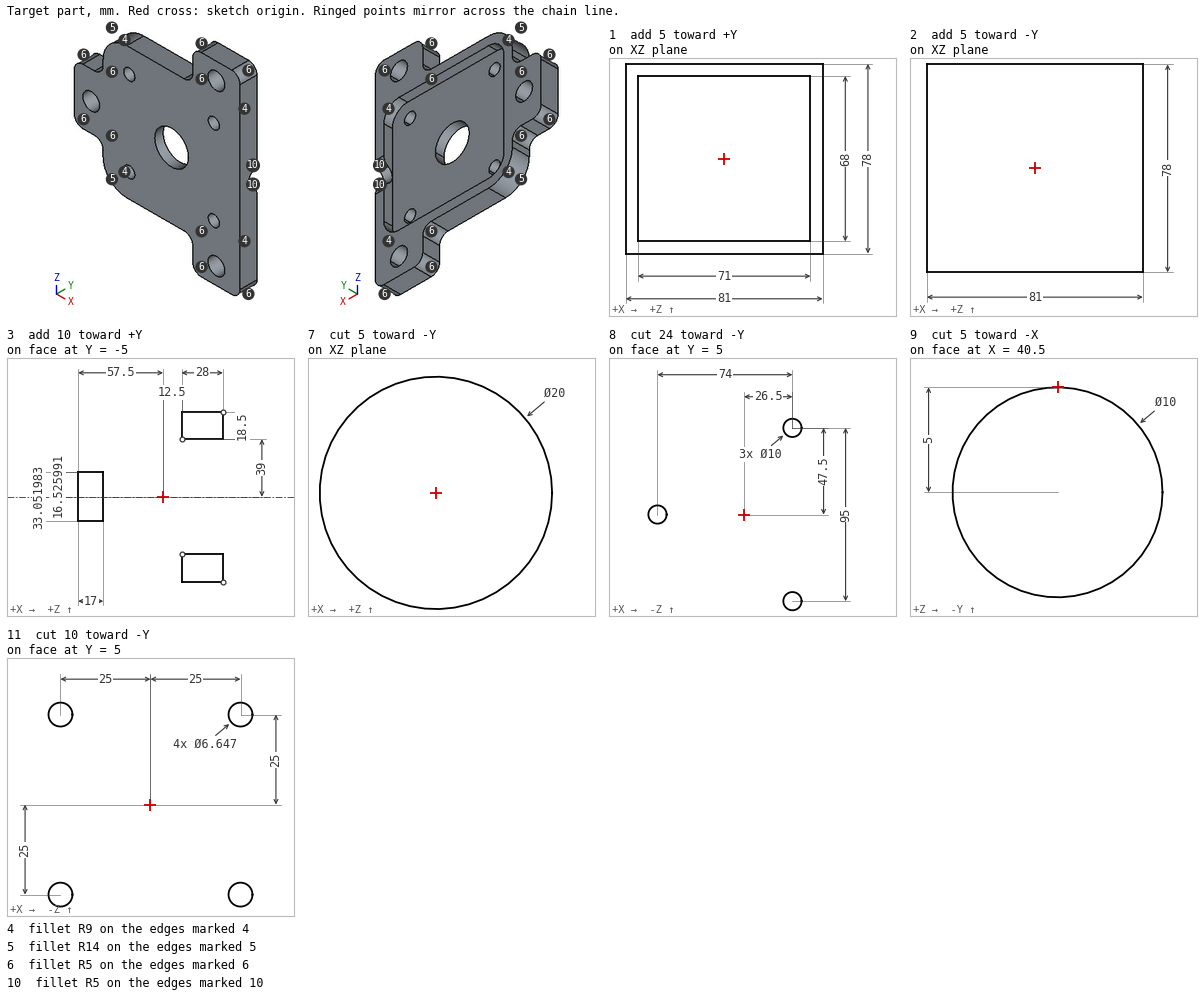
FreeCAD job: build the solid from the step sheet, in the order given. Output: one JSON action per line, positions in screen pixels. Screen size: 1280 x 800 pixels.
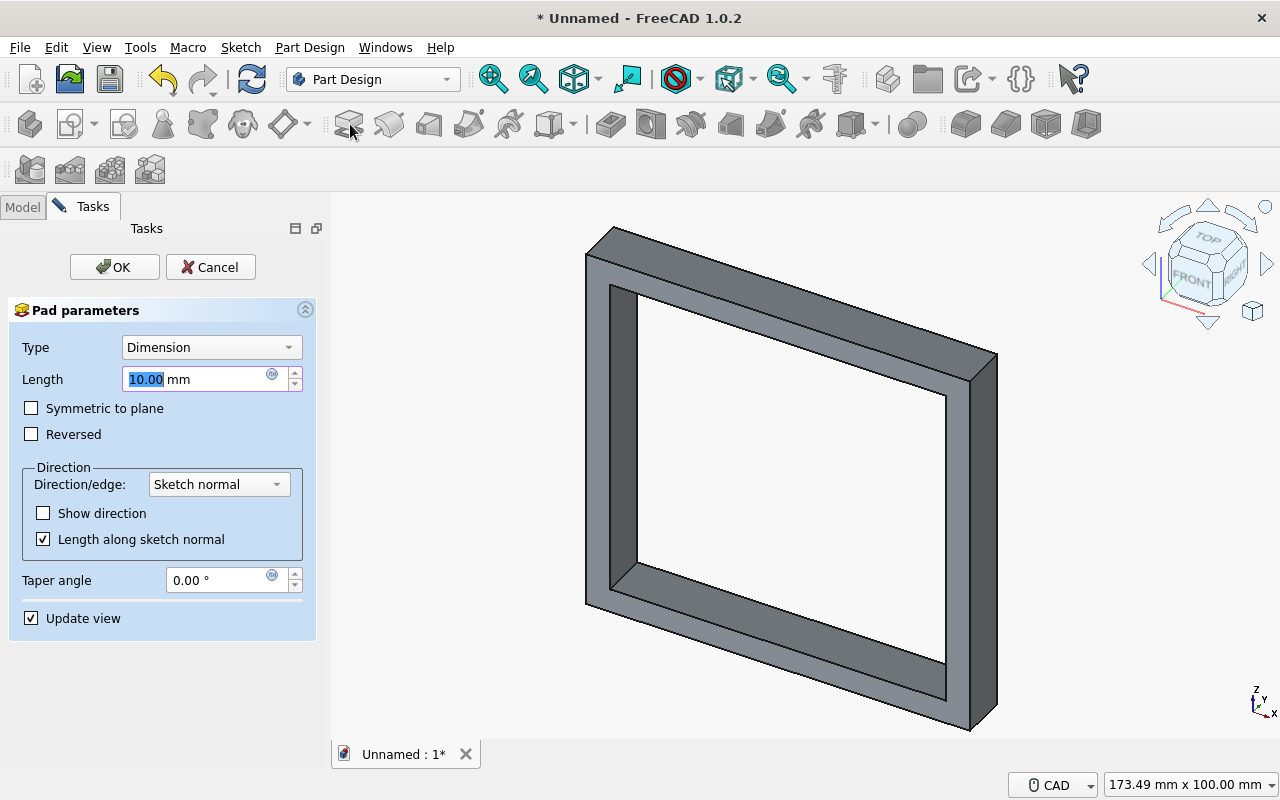
{"action": "type", "text": "5"}
{"action": "key", "text": "Tab"}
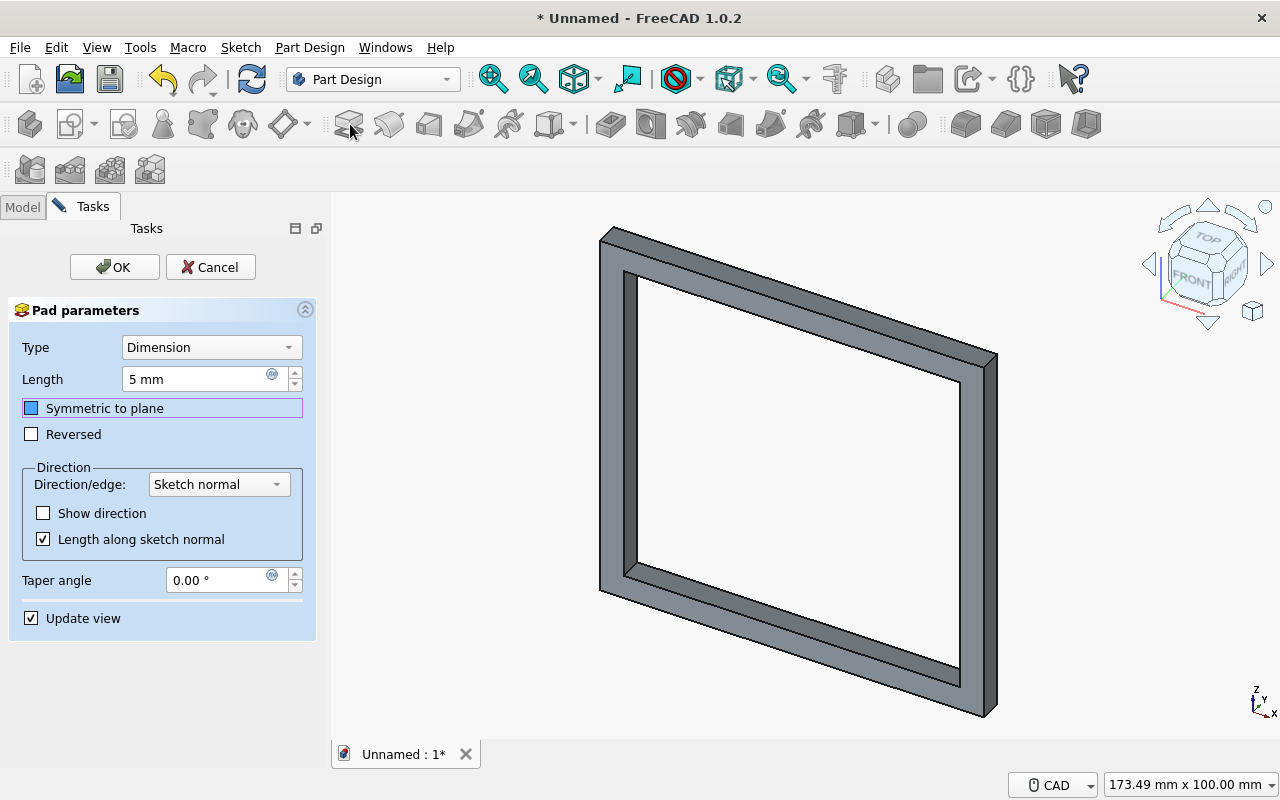
{"action": "left_click", "coordinate": [30, 434]}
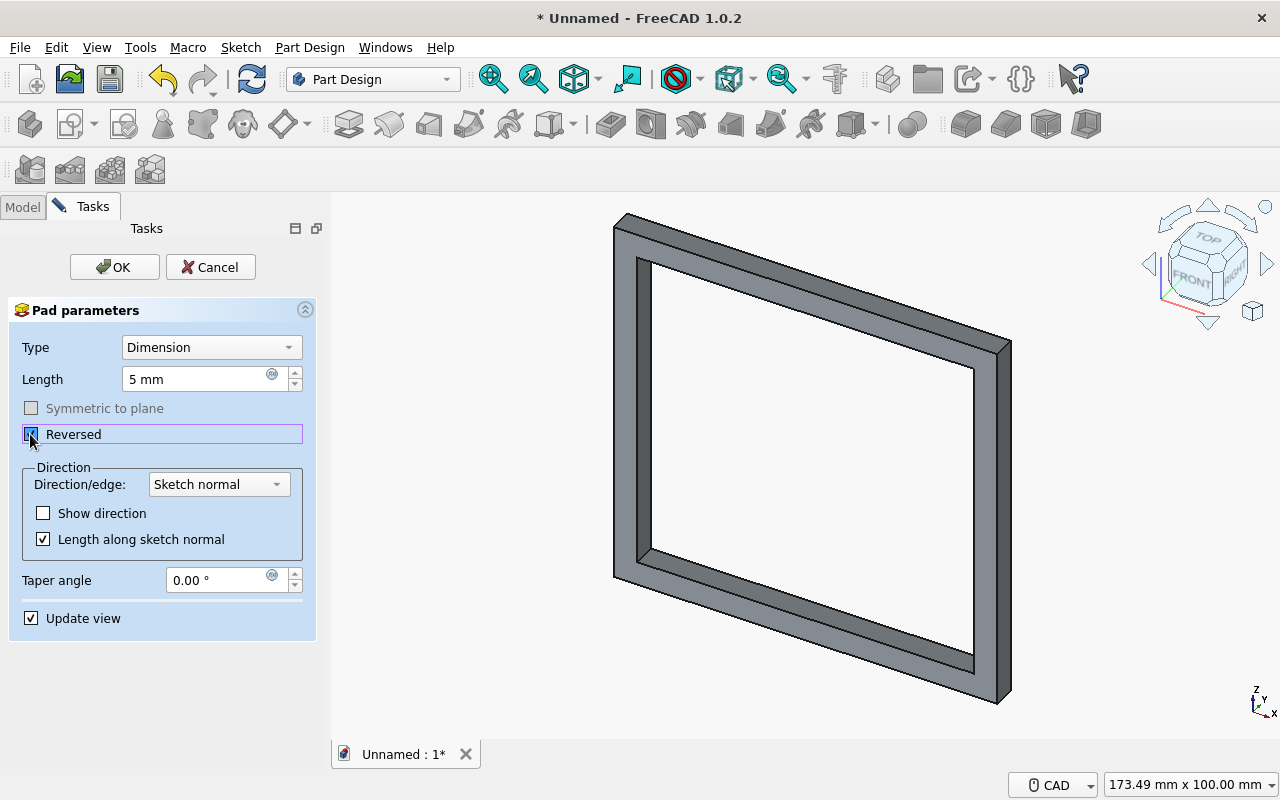
{"action": "left_click", "coordinate": [115, 267]}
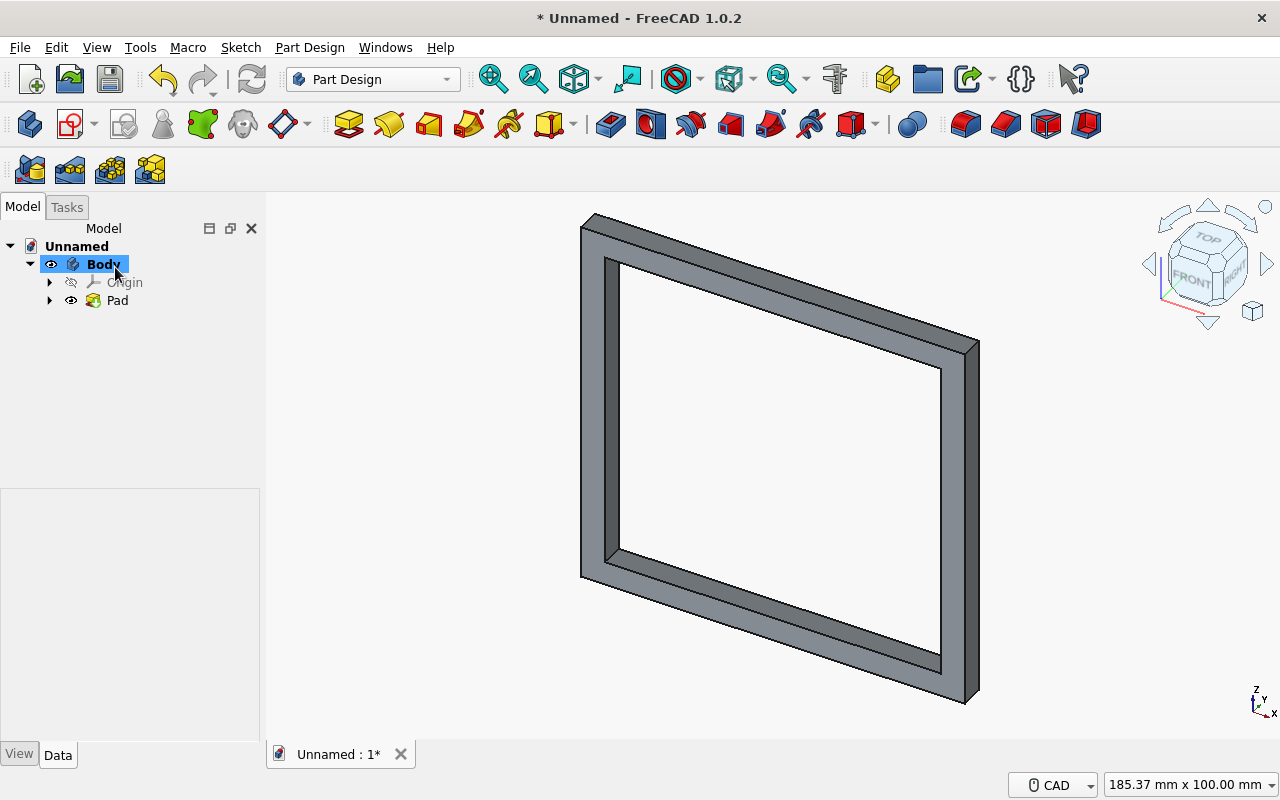
{"action": "left_click", "coordinate": [70, 124]}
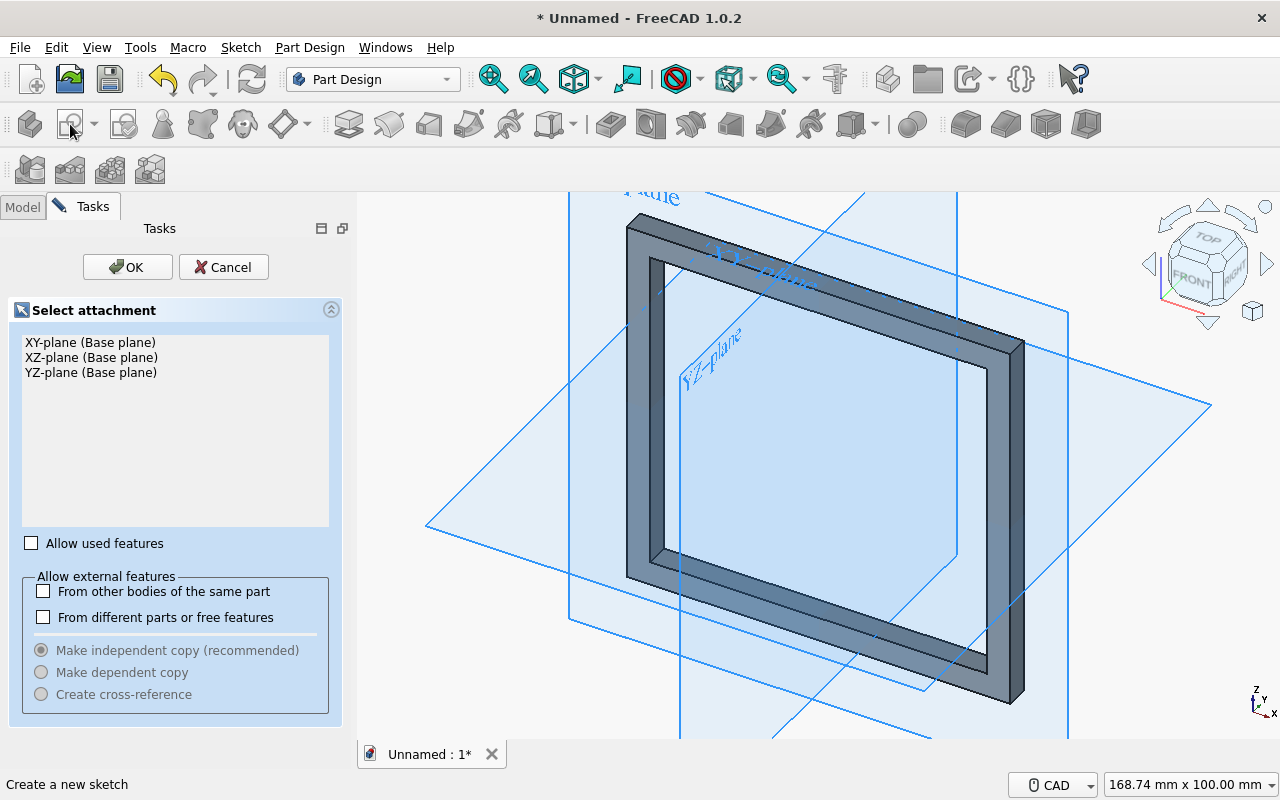
{"action": "left_click", "coordinate": [82, 358]}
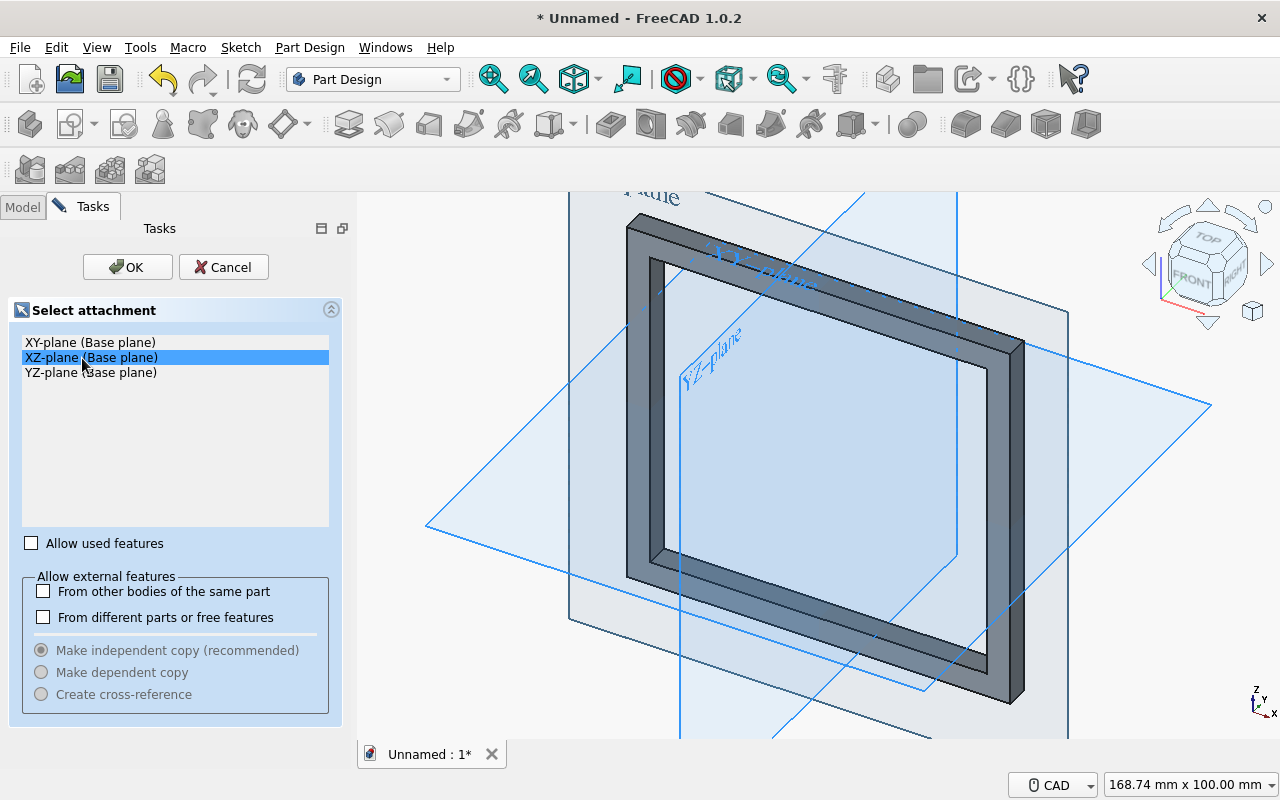
{"action": "left_click", "coordinate": [128, 267]}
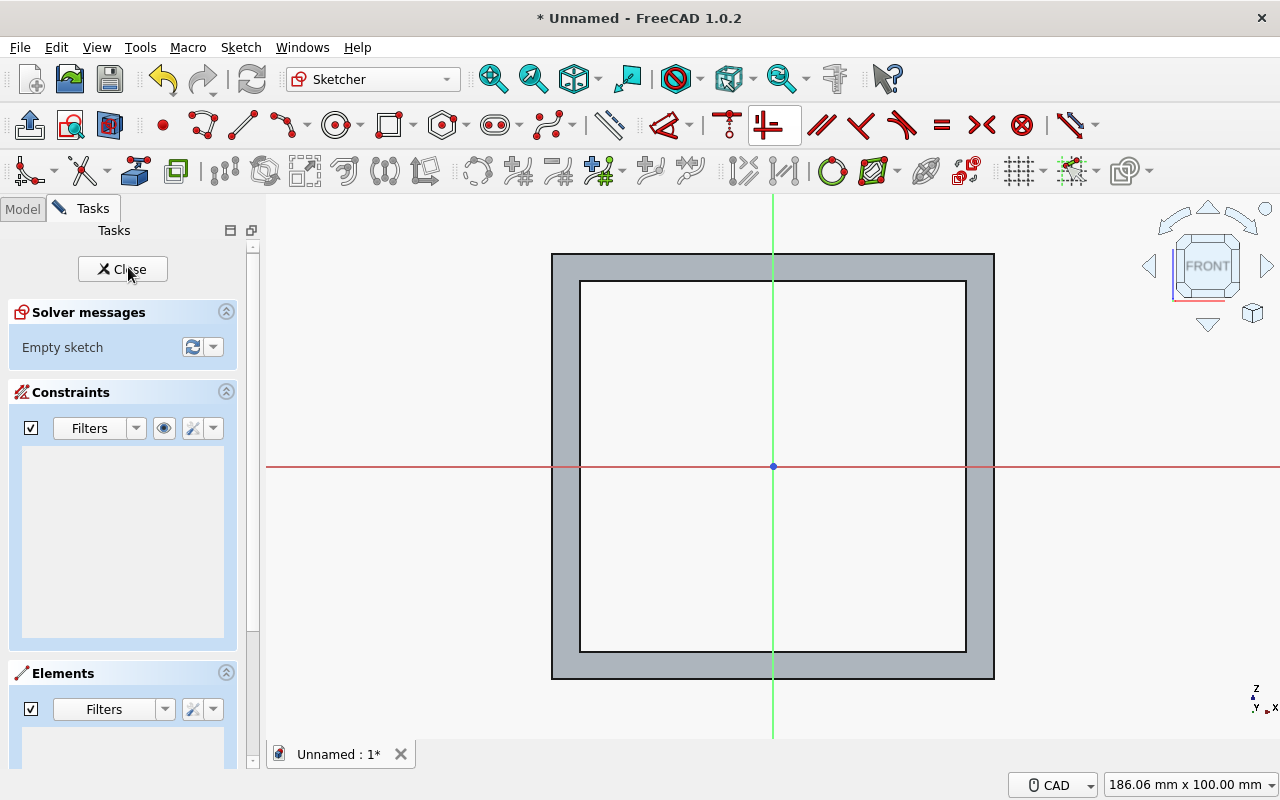
{"action": "key", "text": "g v"}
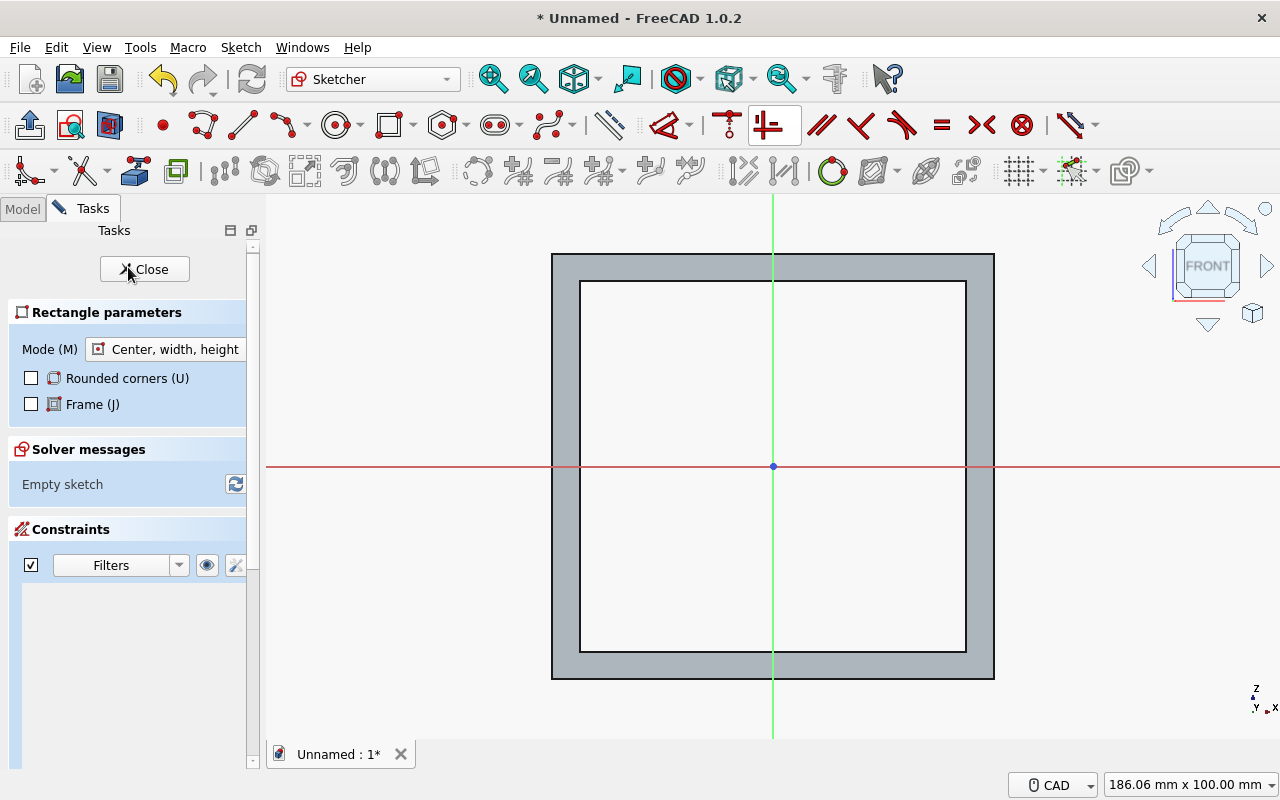
{"action": "left_click", "coordinate": [773, 466]}
{"action": "left_click", "coordinate": [994, 254]}
{"action": "key", "text": "Escape"}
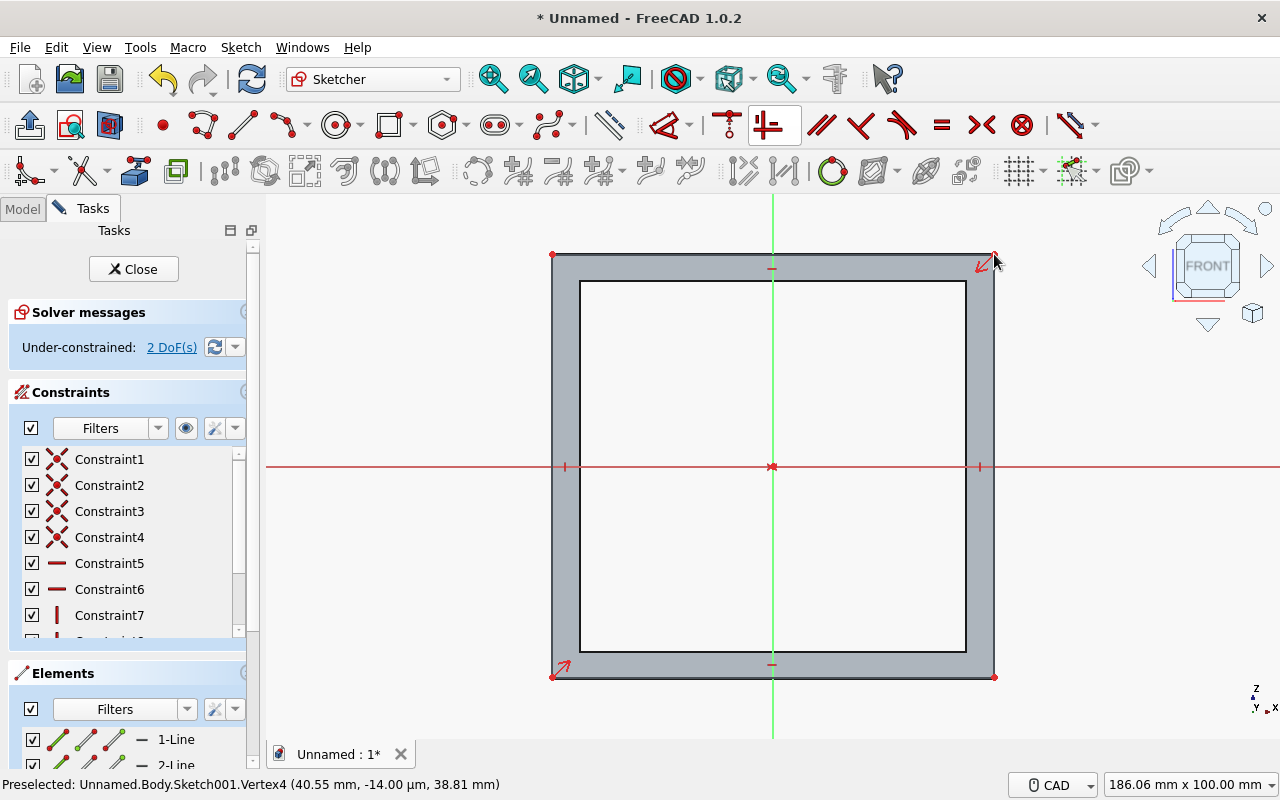
{"action": "key", "text": "d"}